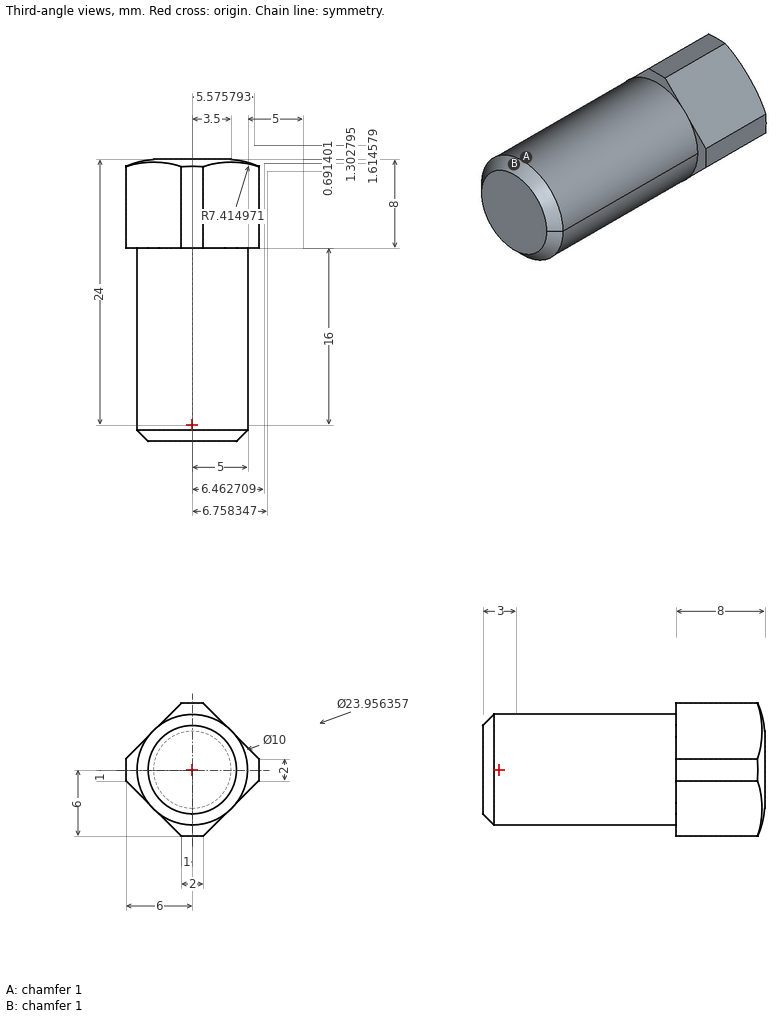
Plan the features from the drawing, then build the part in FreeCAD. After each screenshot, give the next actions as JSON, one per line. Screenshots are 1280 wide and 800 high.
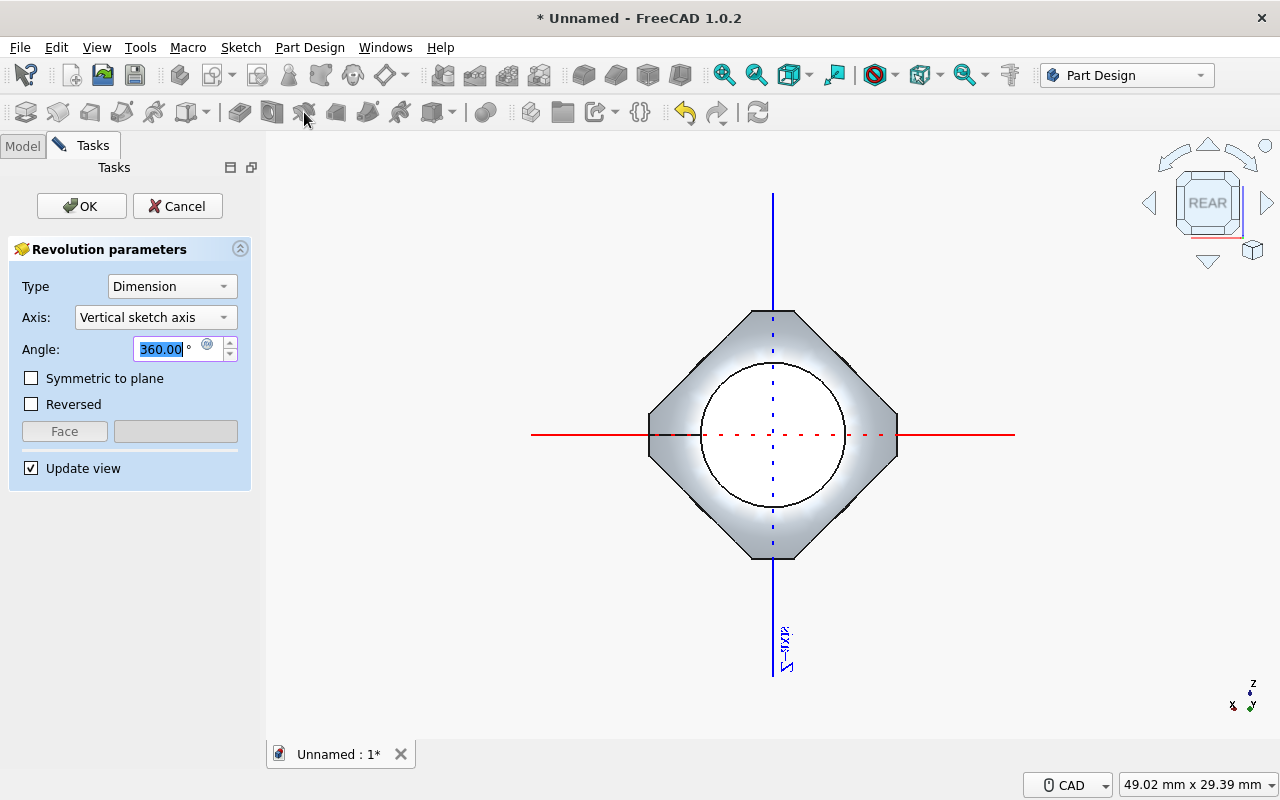
{"action": "left_click", "coordinate": [82, 206]}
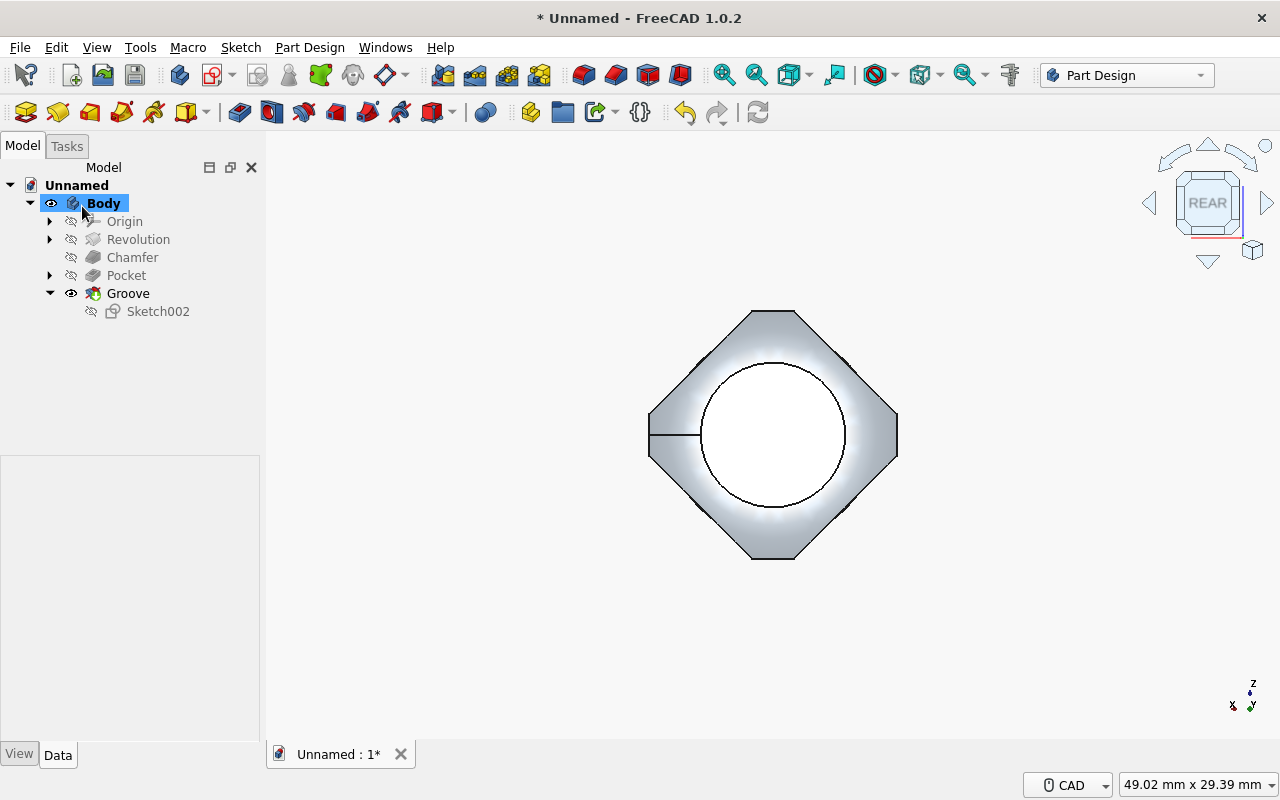
{"action": "left_click", "coordinate": [726, 76]}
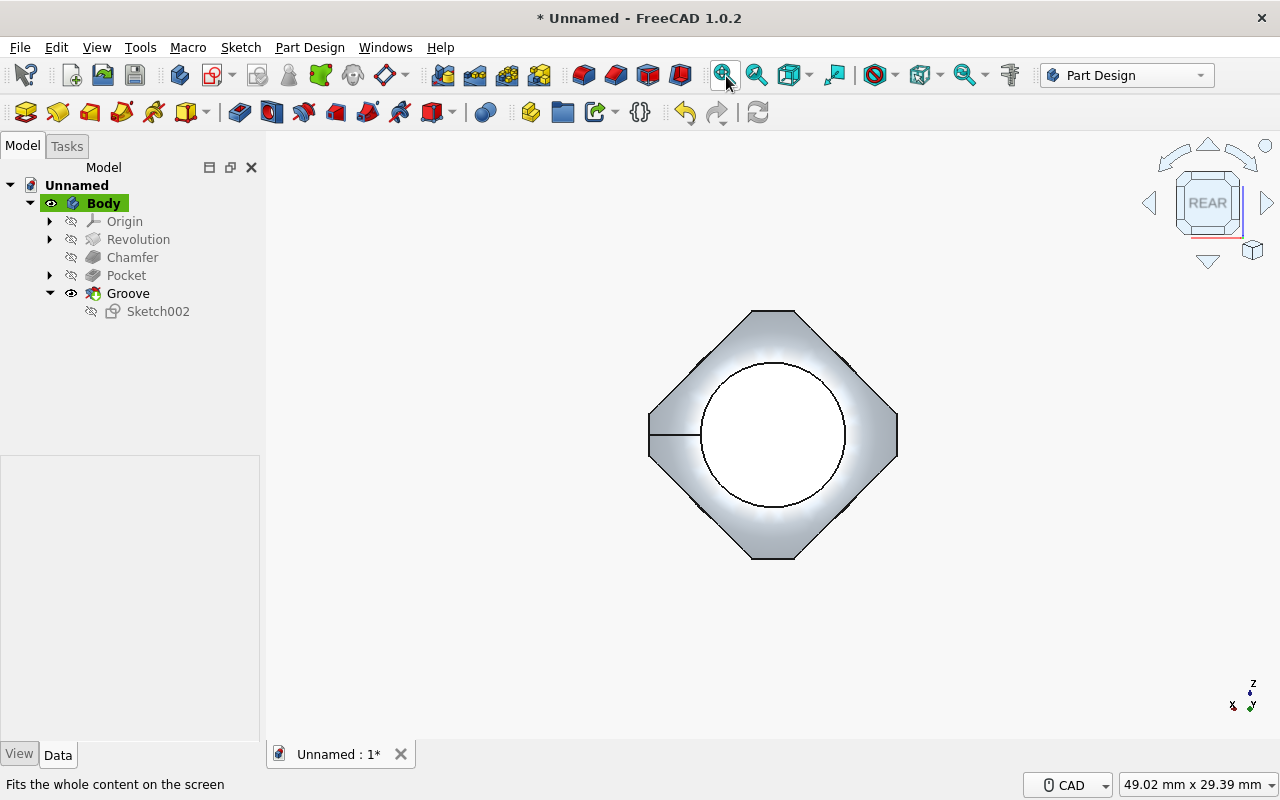
{"action": "key", "text": "0"}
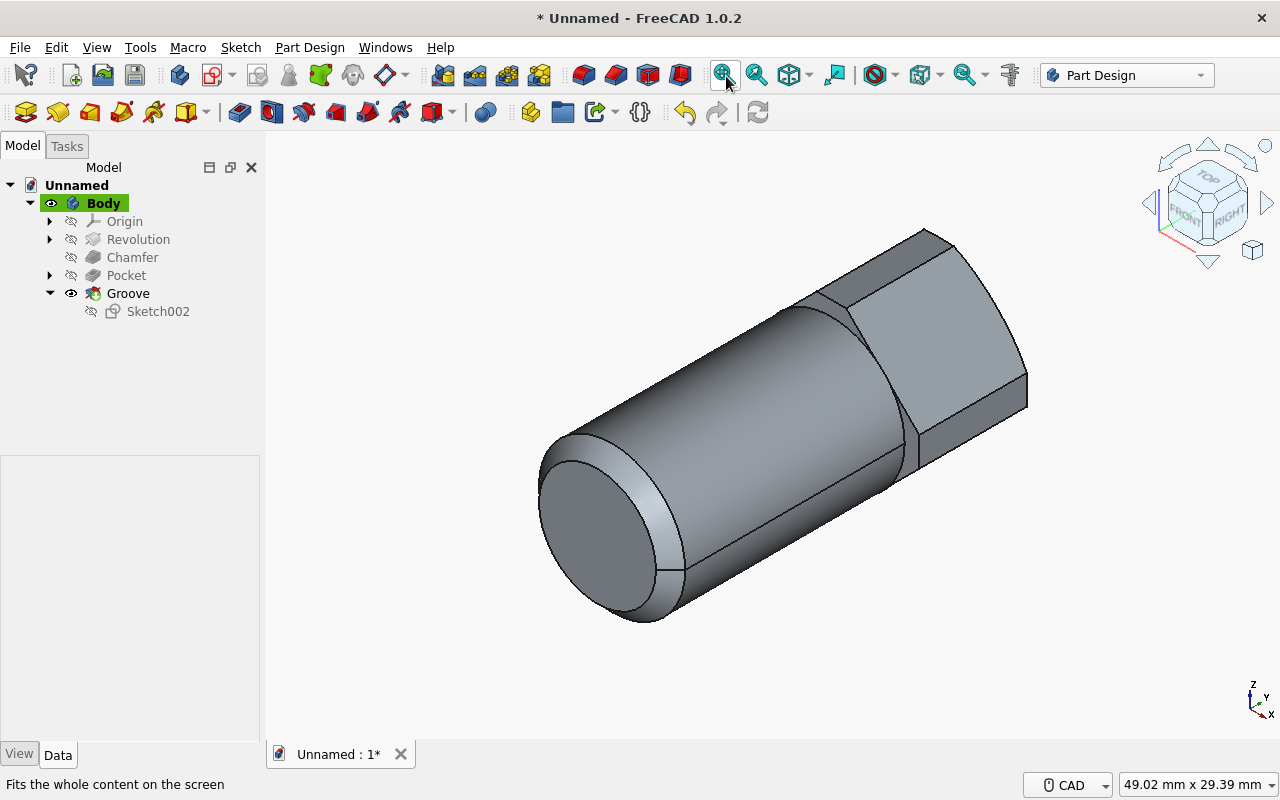
{"action": "left_click", "coordinate": [597, 535]}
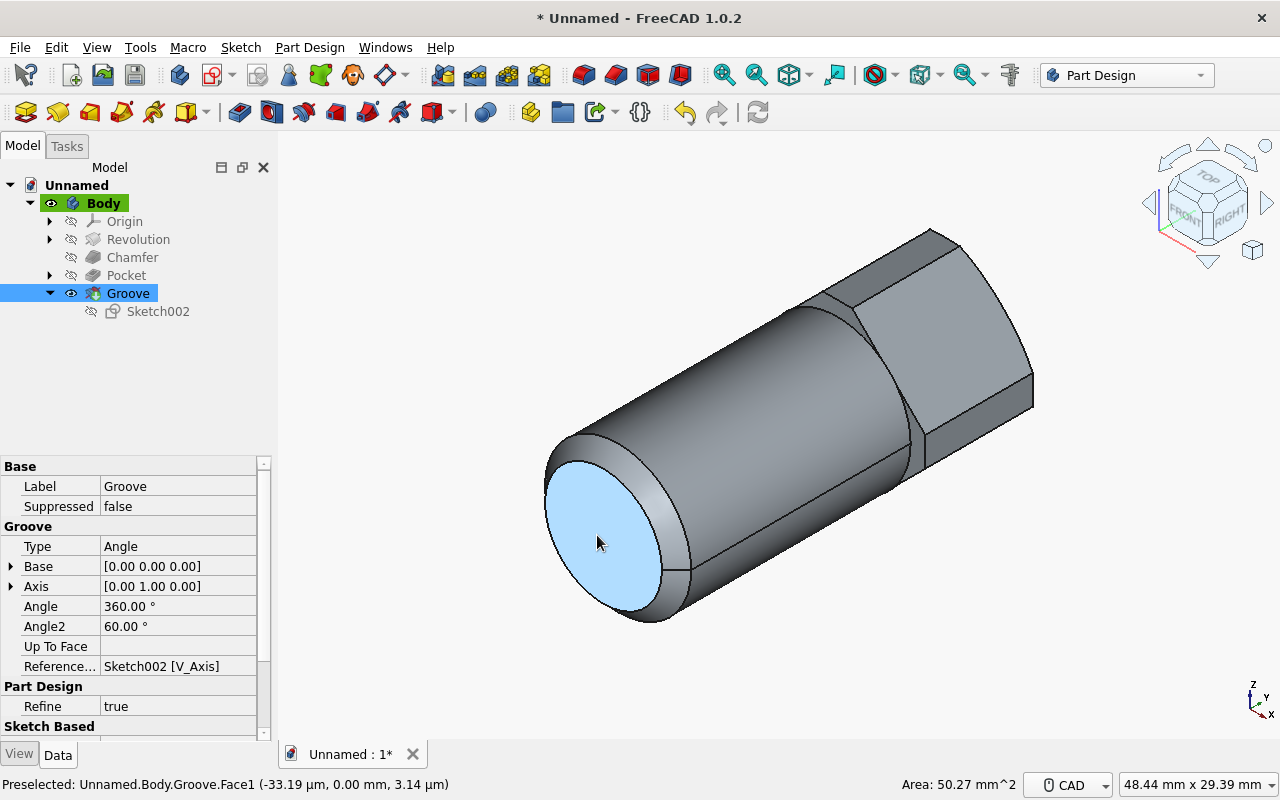
{"action": "left_click", "coordinate": [212, 76]}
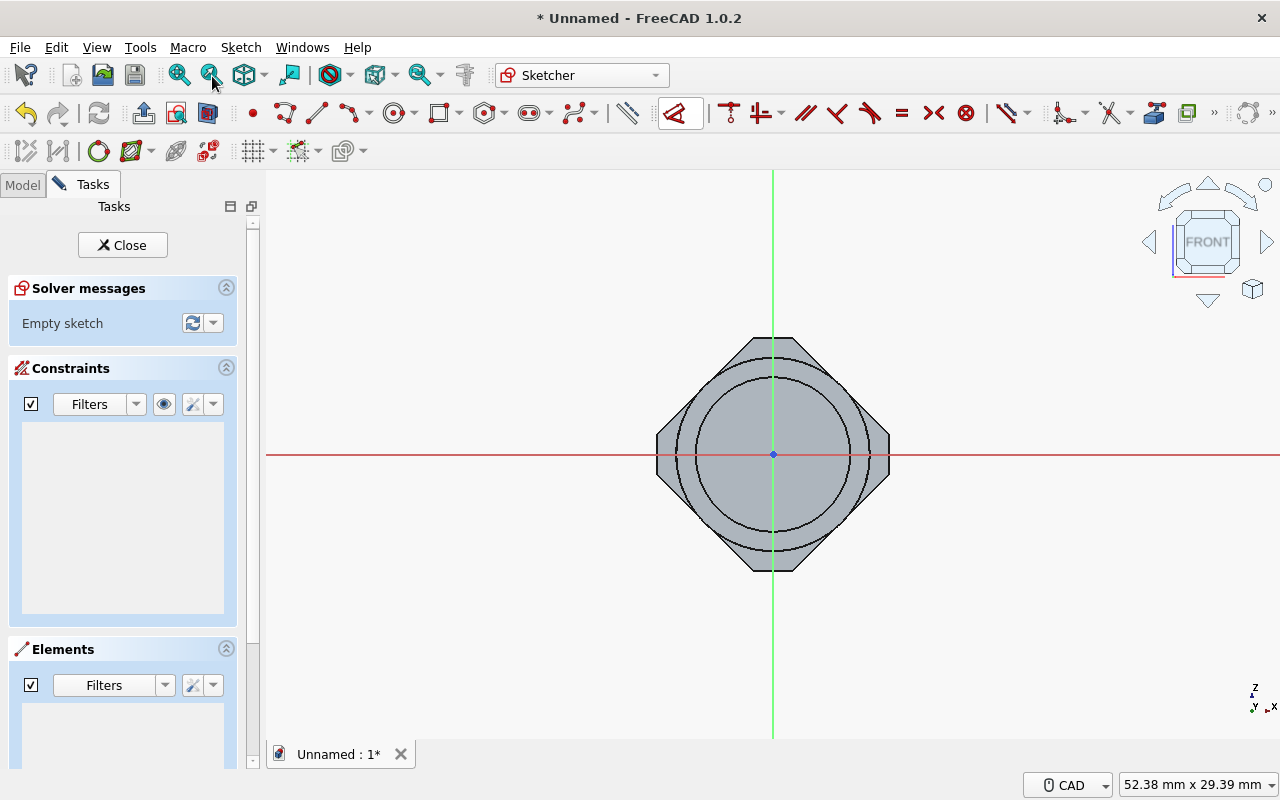
{"action": "scroll", "coordinate": [856, 455], "scroll_direction": "up", "scroll_amount": 3}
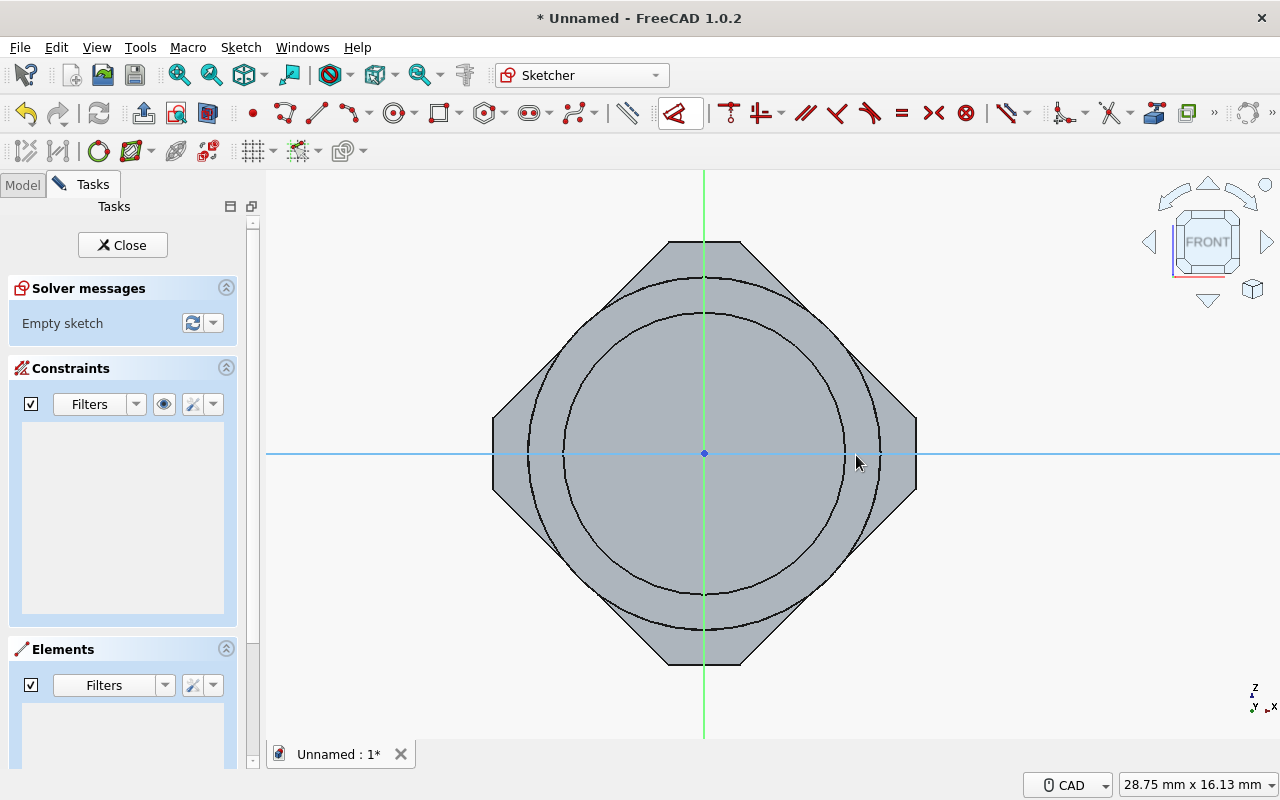
{"action": "left_click", "coordinate": [394, 114]}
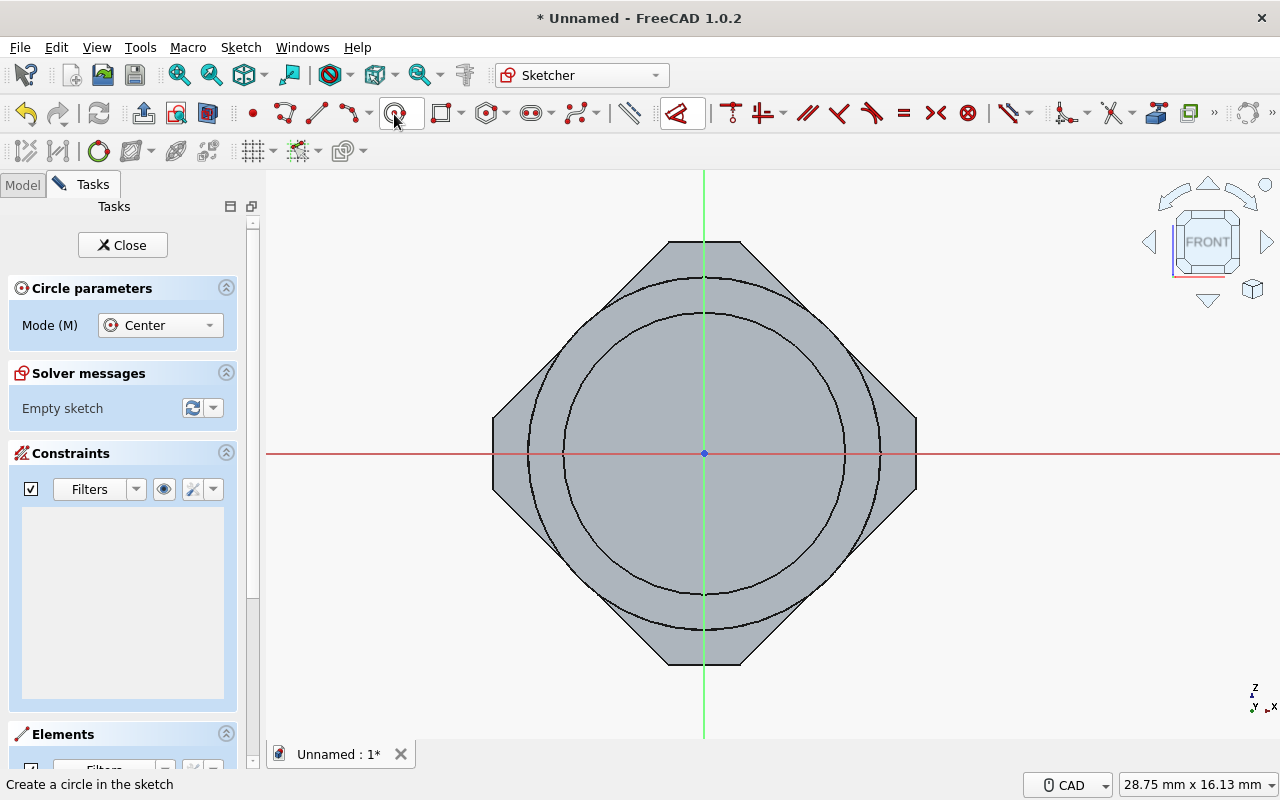
{"action": "left_click", "coordinate": [704, 454]}
{"action": "left_click", "coordinate": [829, 329]}
{"action": "key", "text": "Escape"}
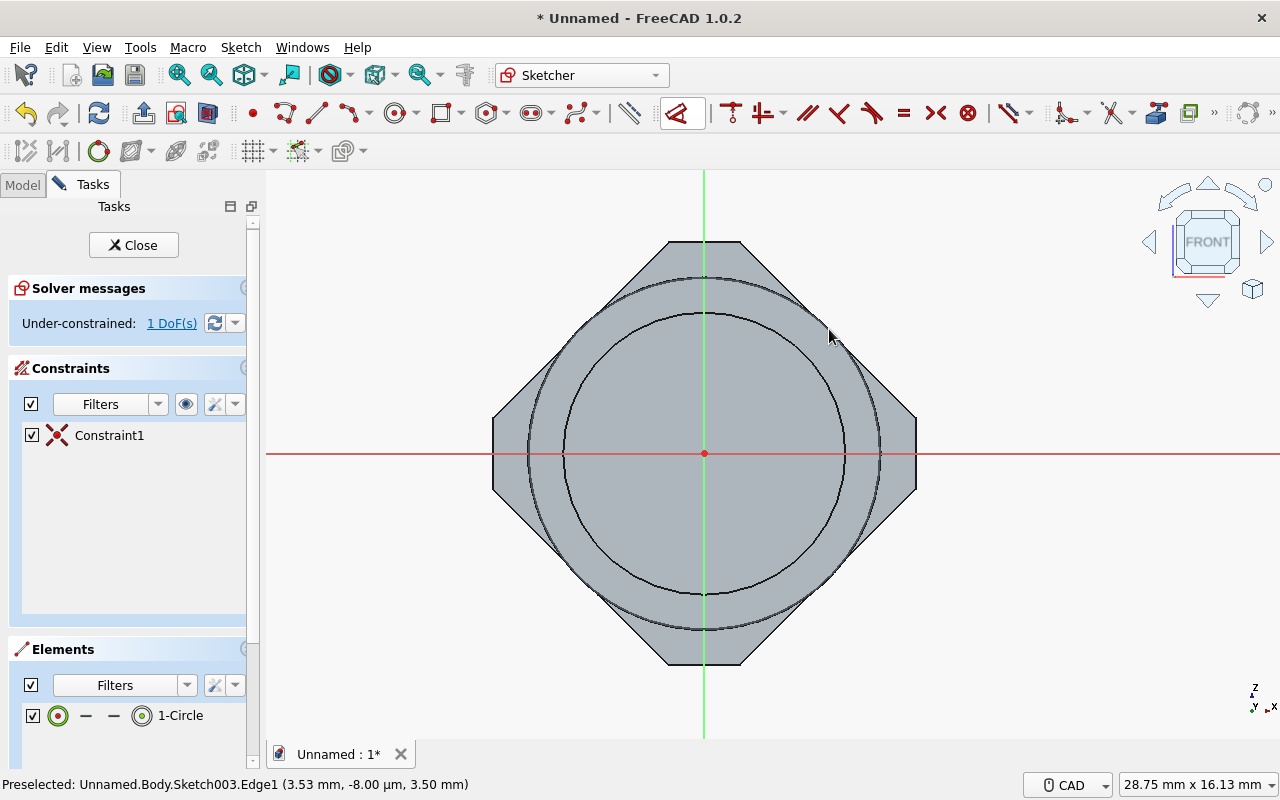
{"action": "left_click", "coordinate": [828, 329]}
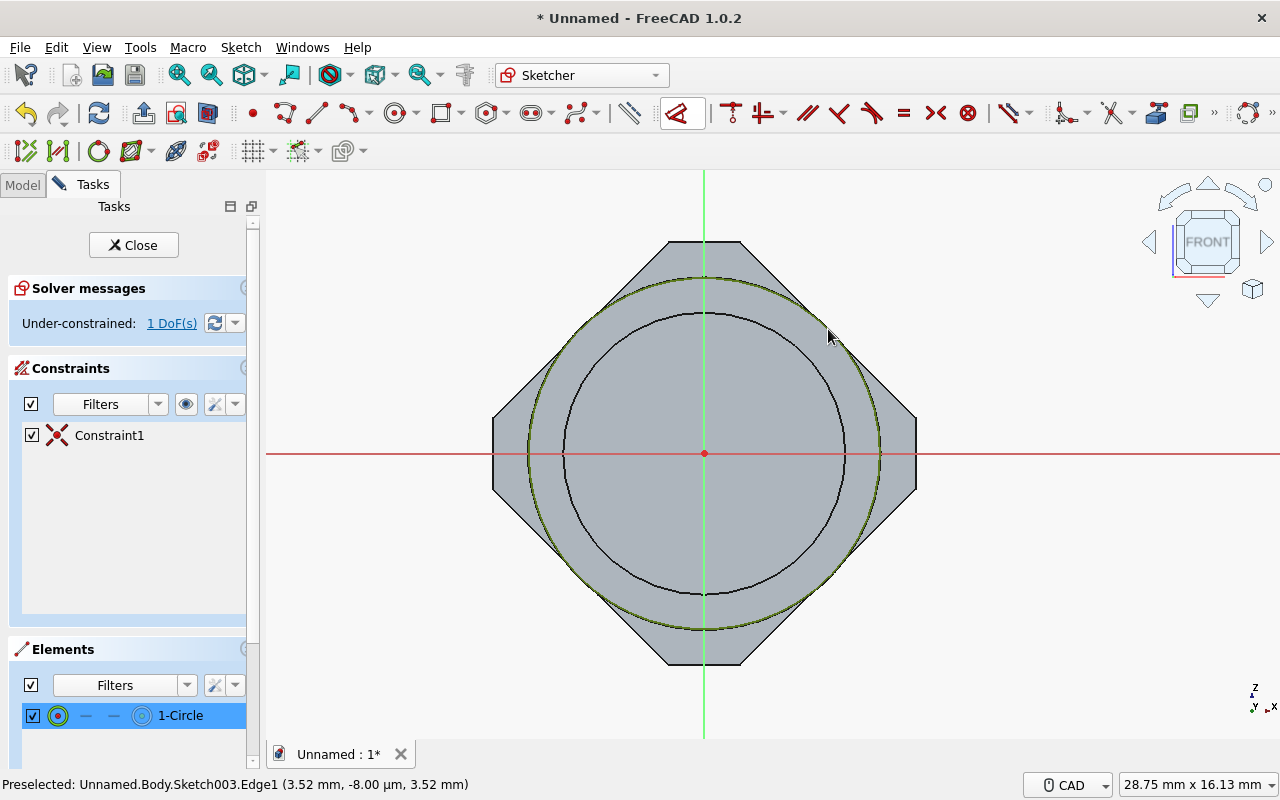
{"action": "left_click", "coordinate": [700, 114]}